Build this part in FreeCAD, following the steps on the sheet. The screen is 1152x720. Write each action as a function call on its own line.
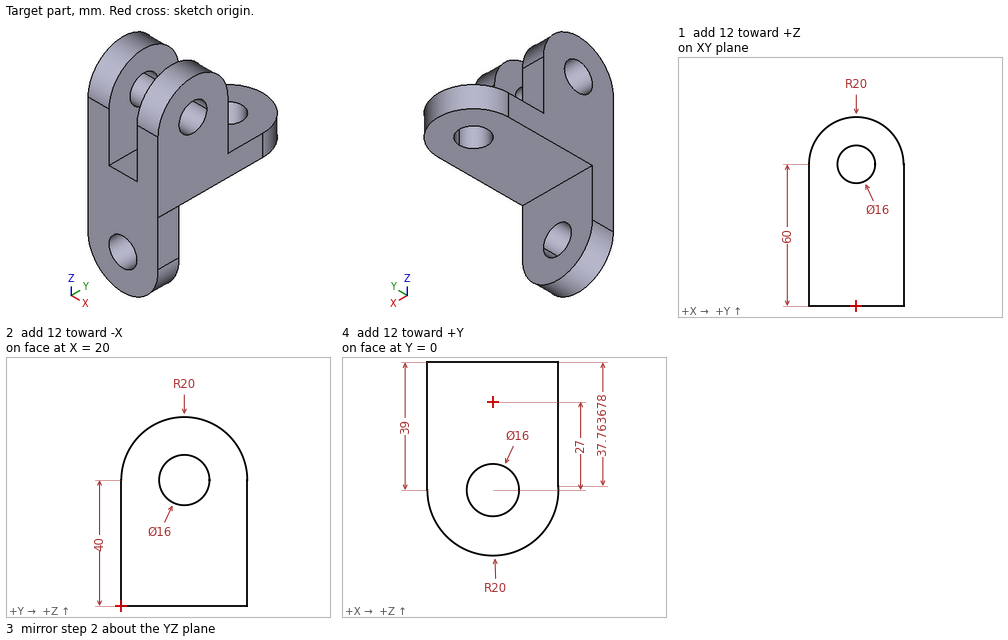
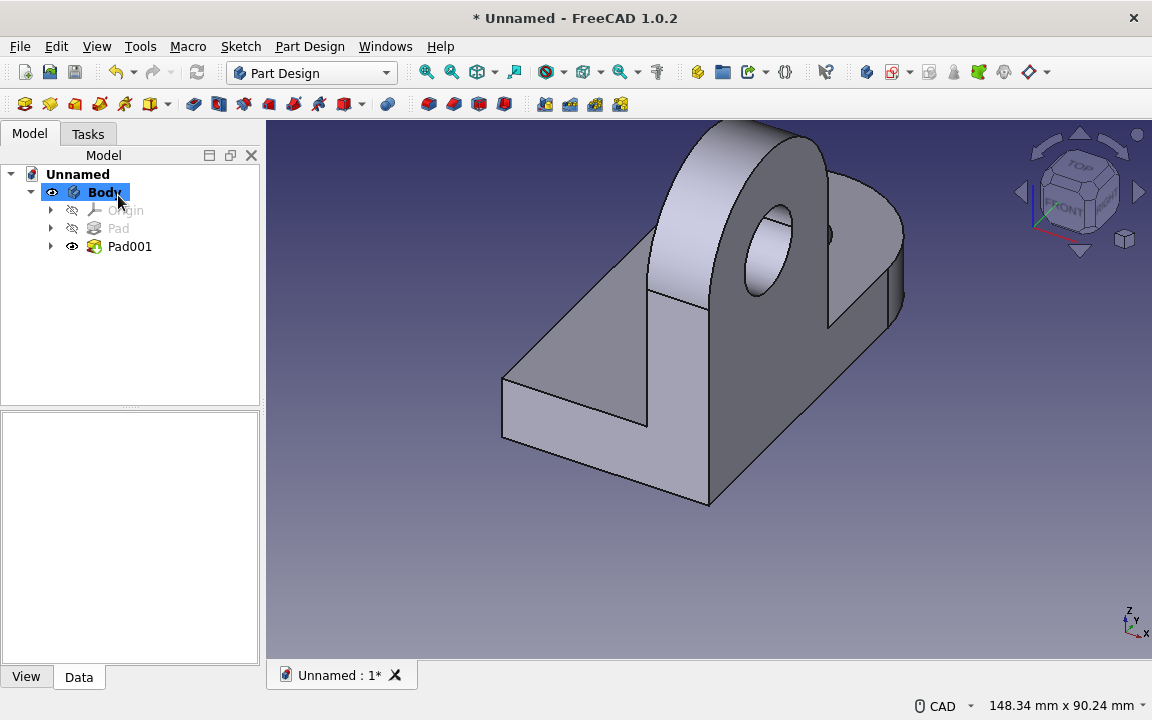
key(v)
key(f)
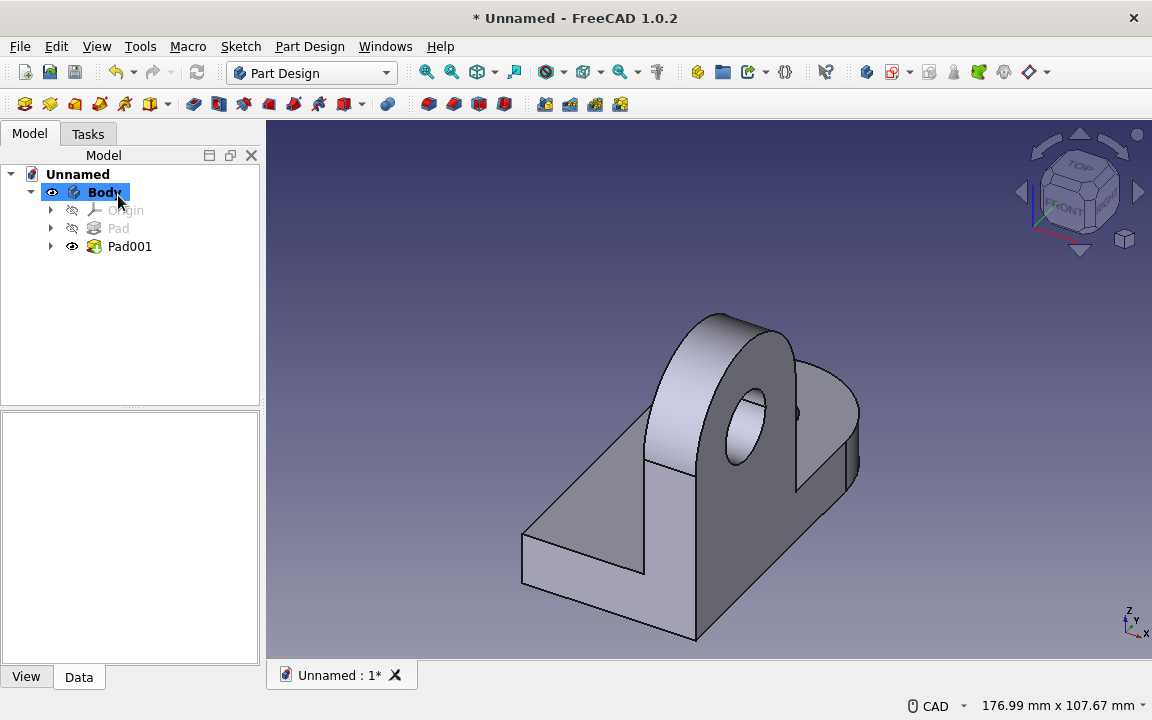
click(117, 246)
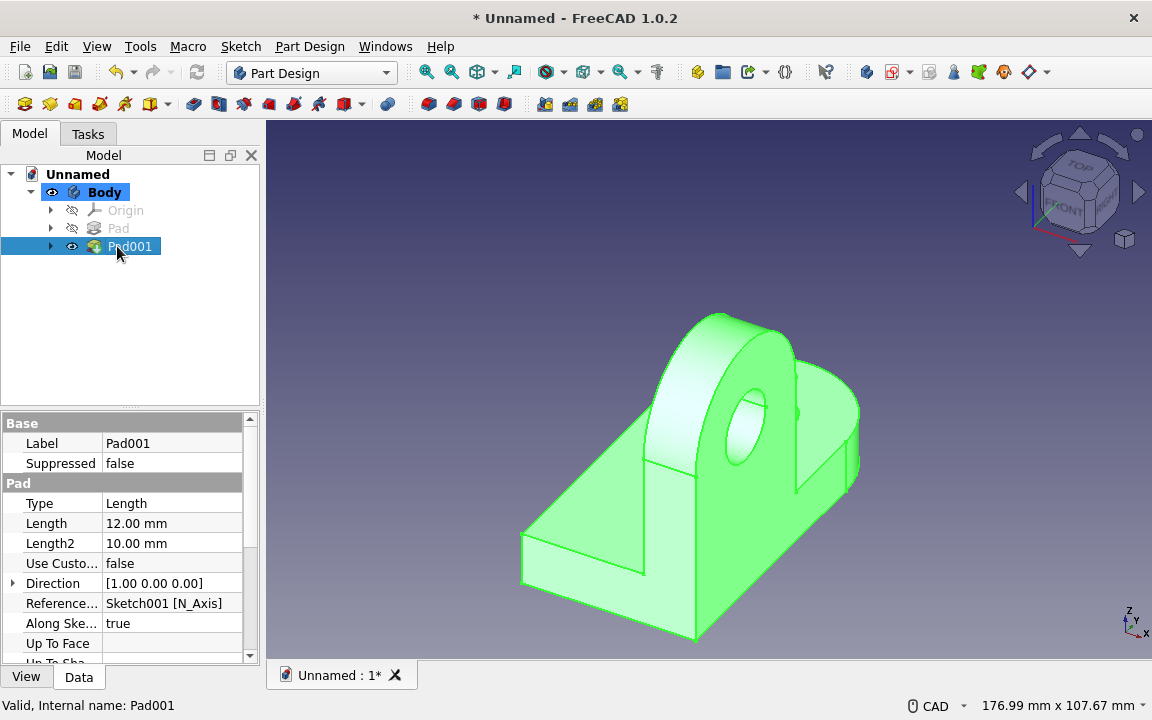
click(545, 104)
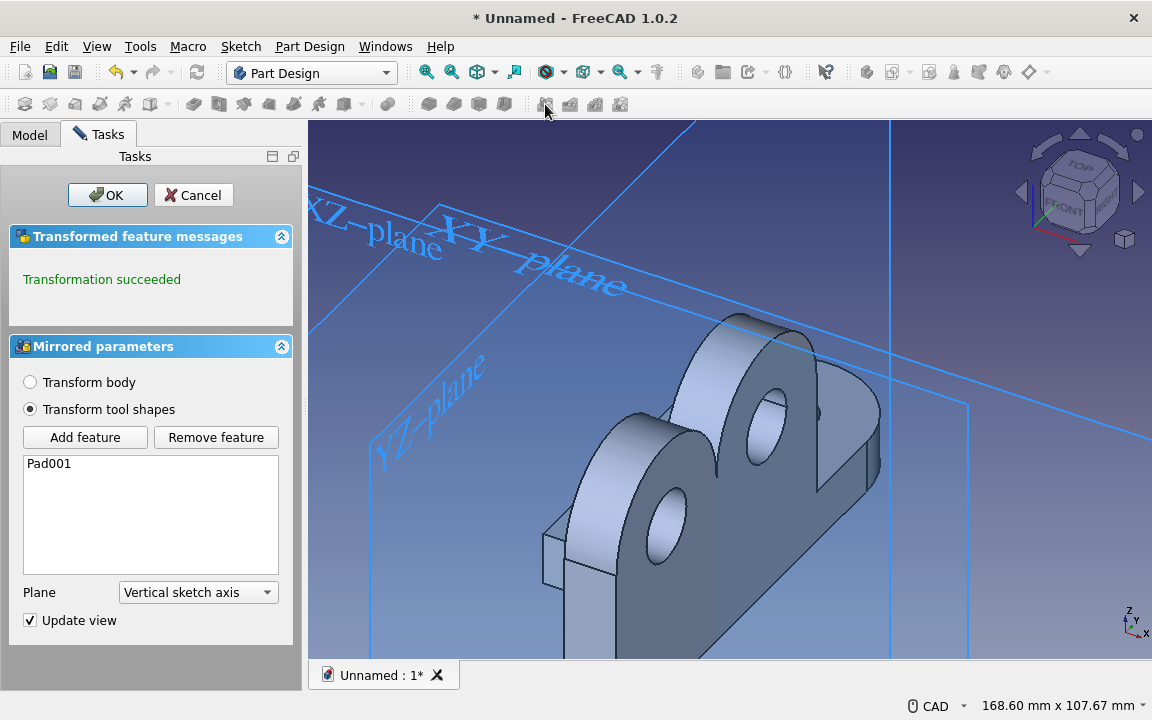
click(199, 592)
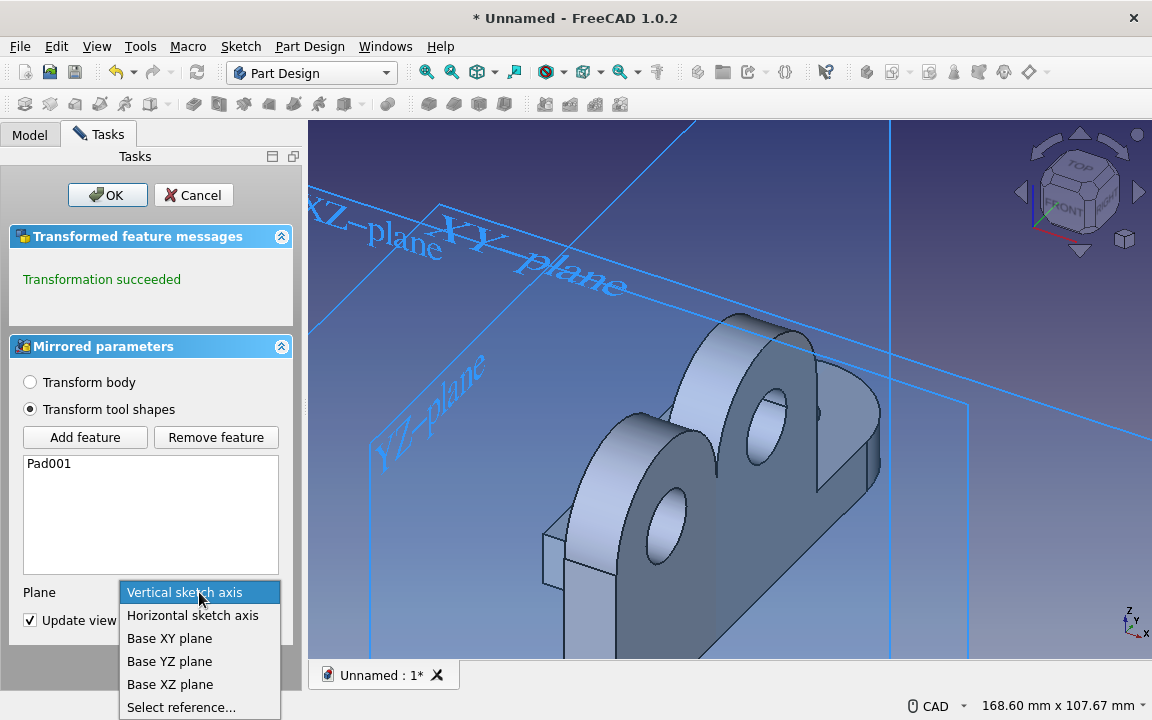
click(198, 662)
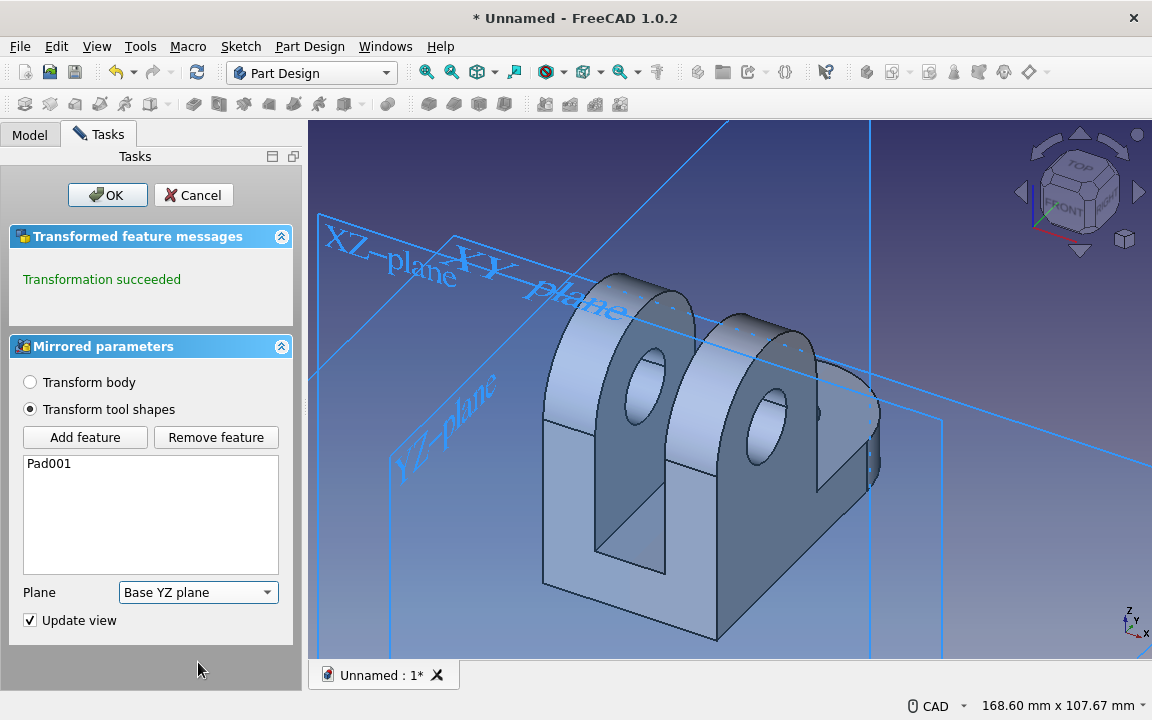
click(108, 195)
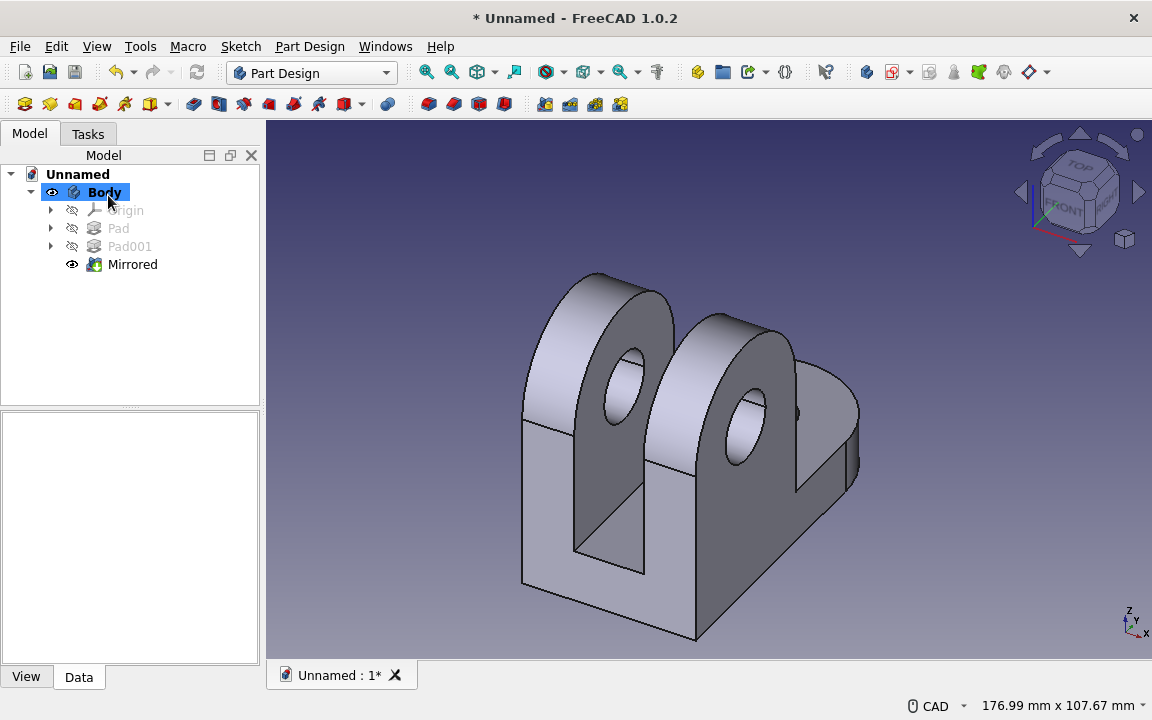
click(559, 559)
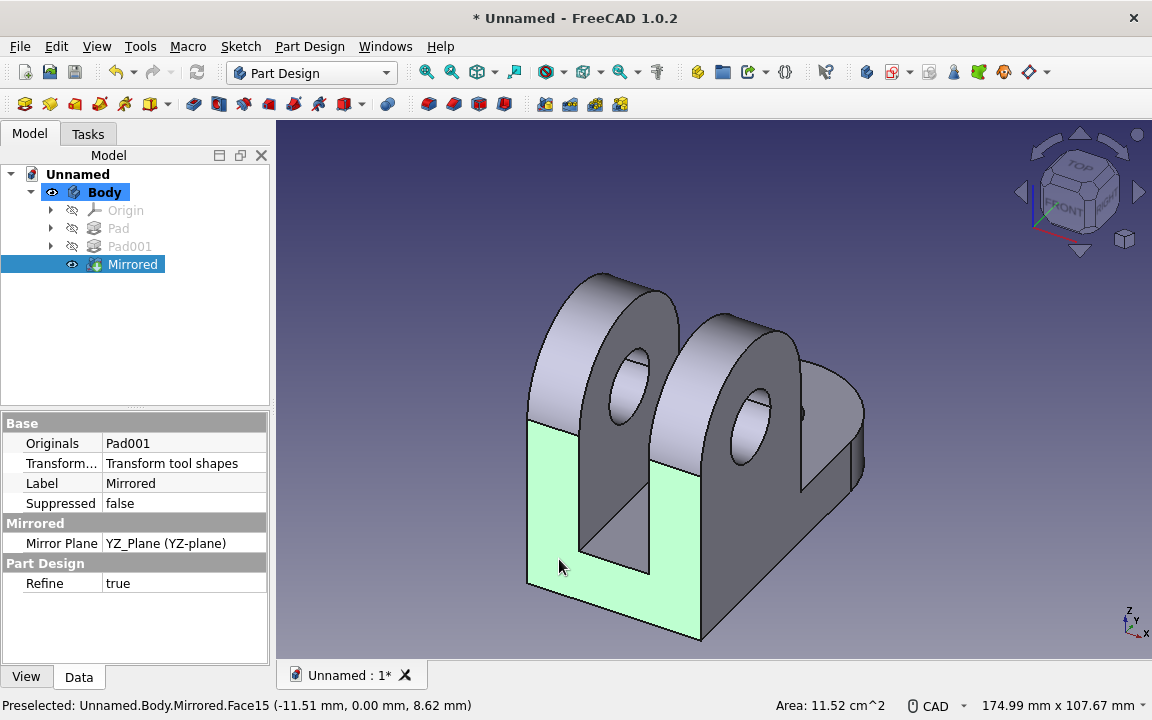
click(892, 72)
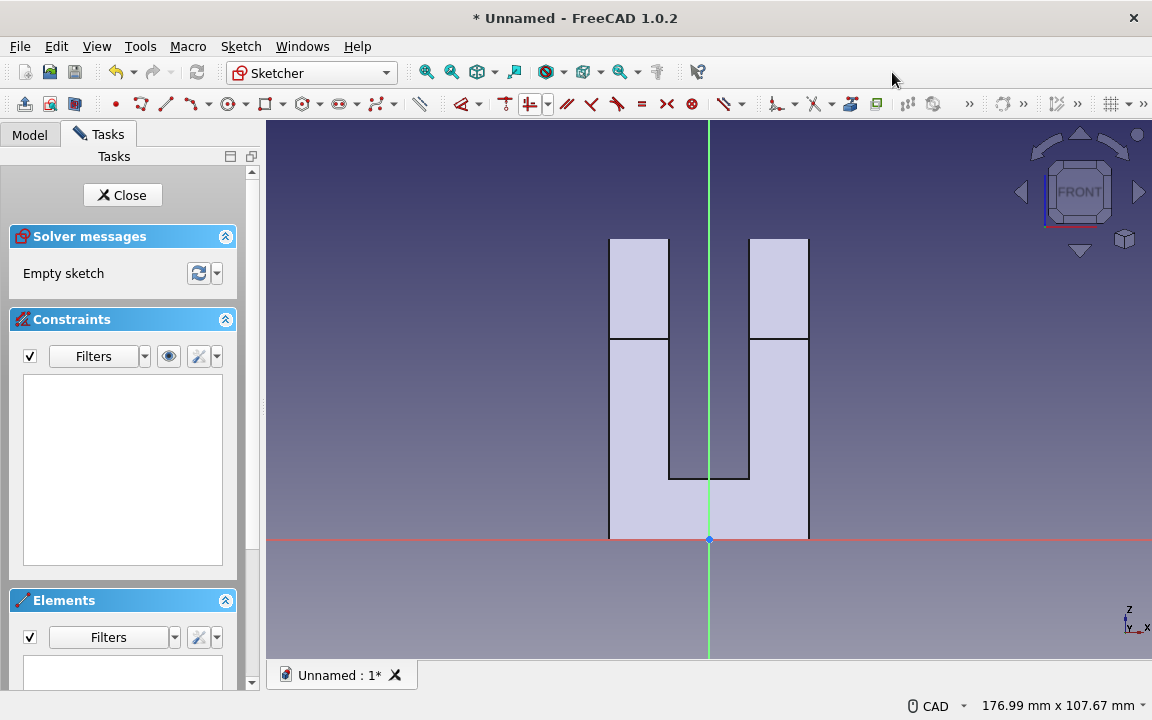
scroll(501, 148, down, 2)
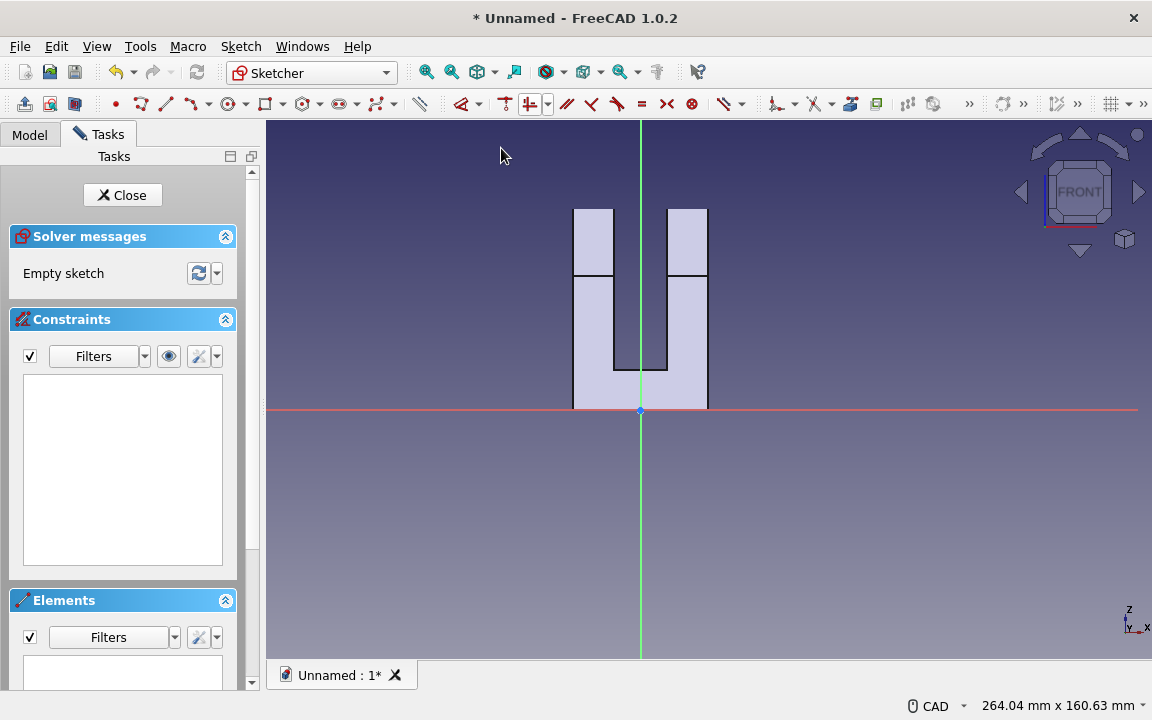
scroll(640, 566, up, 3)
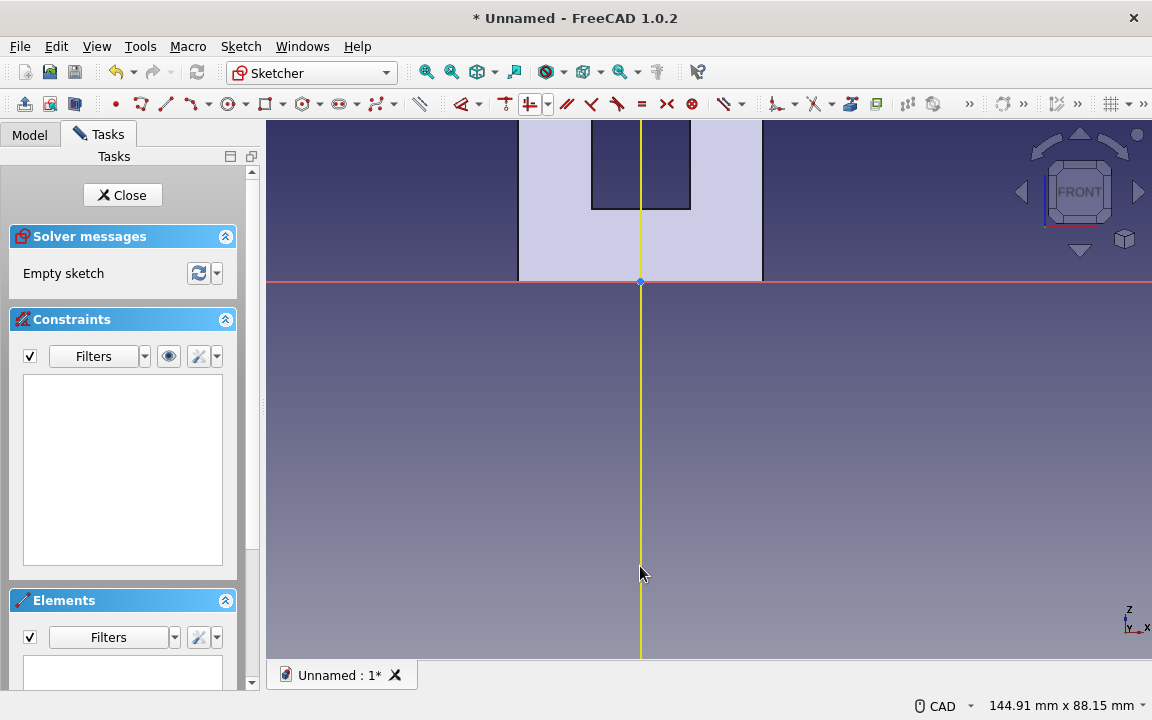
key(g)
key(m)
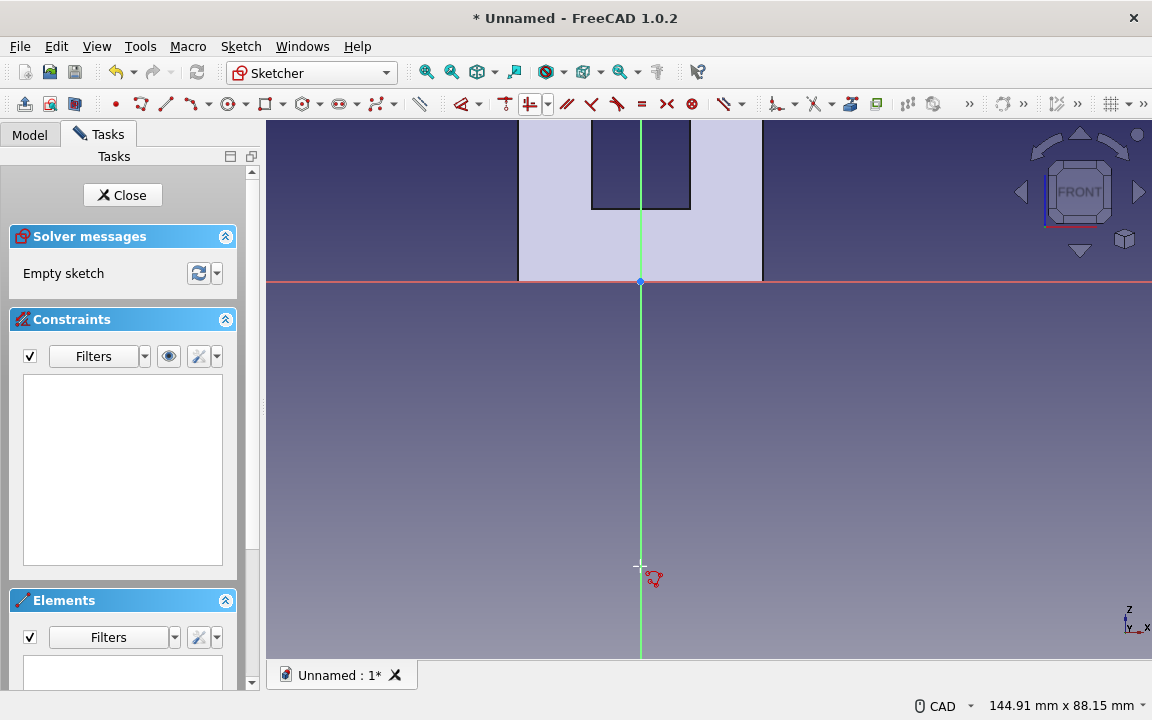
click(763, 439)
click(763, 209)
click(518, 209)
click(518, 447)
right_click(518, 447)